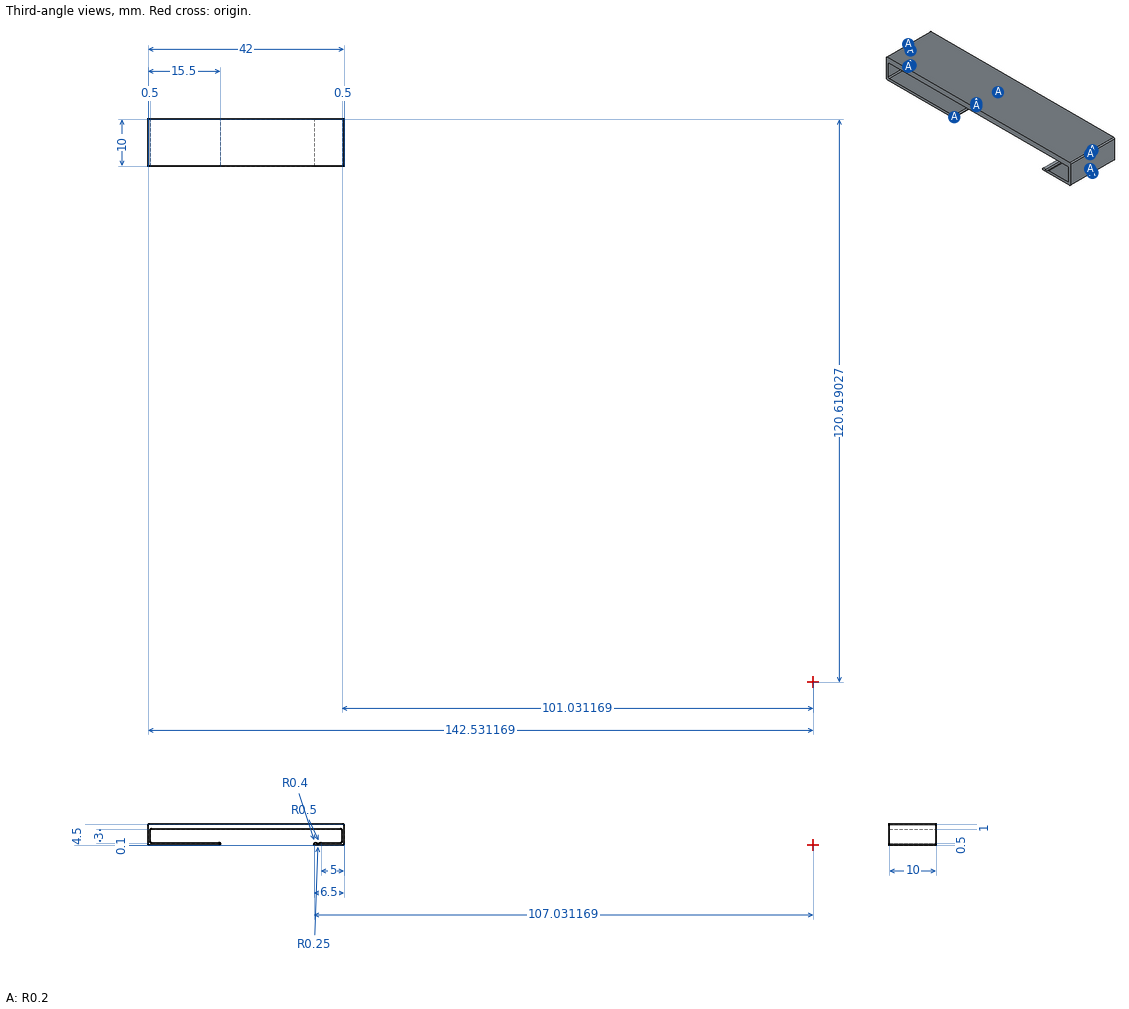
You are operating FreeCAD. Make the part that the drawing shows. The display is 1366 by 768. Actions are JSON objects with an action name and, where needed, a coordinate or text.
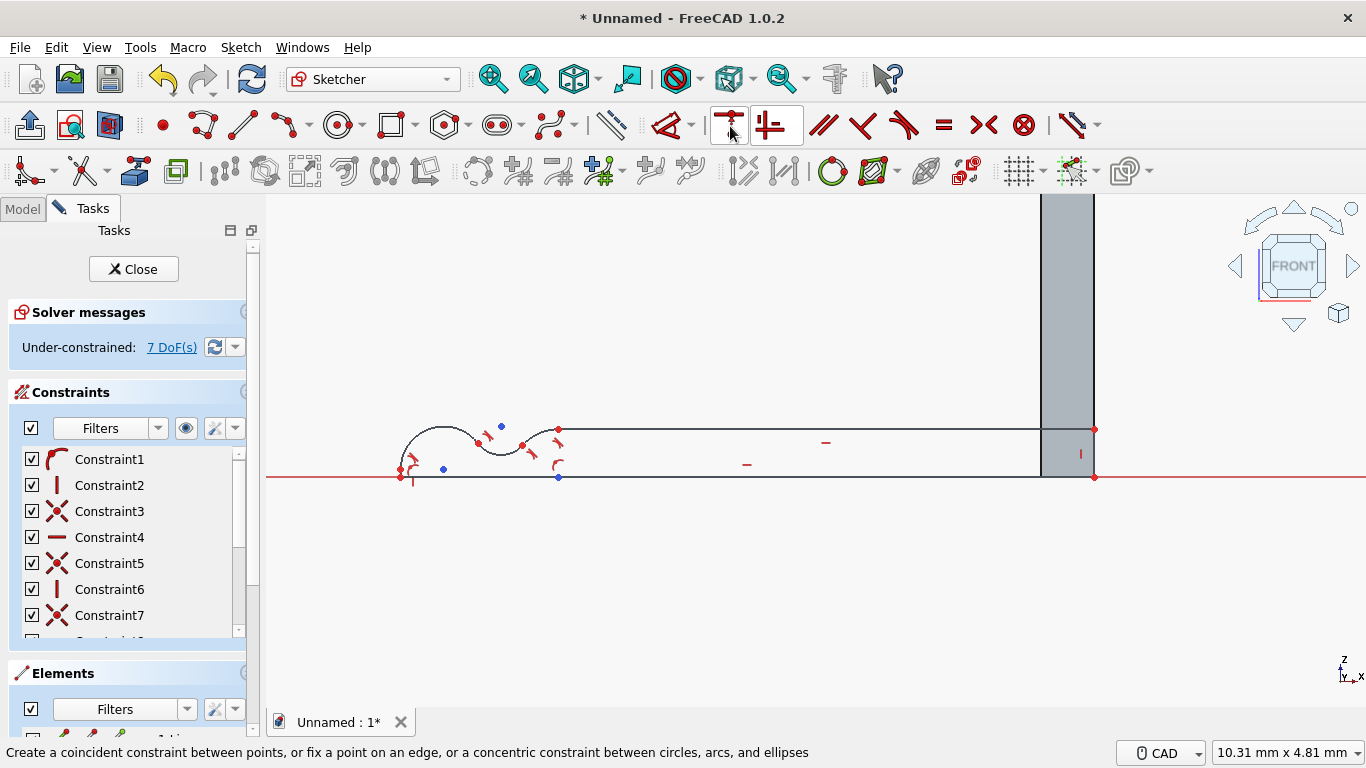
{"action": "left_click", "coordinate": [666, 126]}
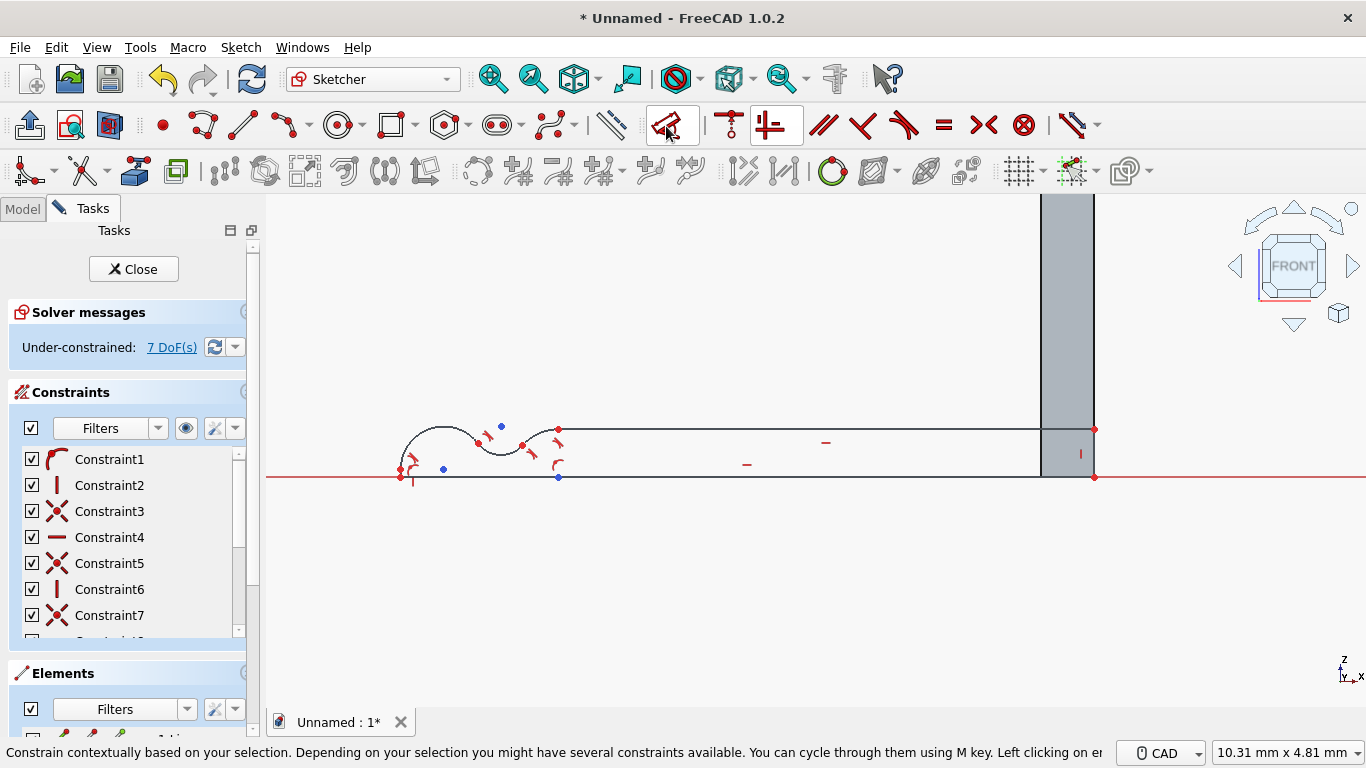
{"action": "left_click", "coordinate": [546, 431]}
{"action": "left_click", "coordinate": [538, 400]}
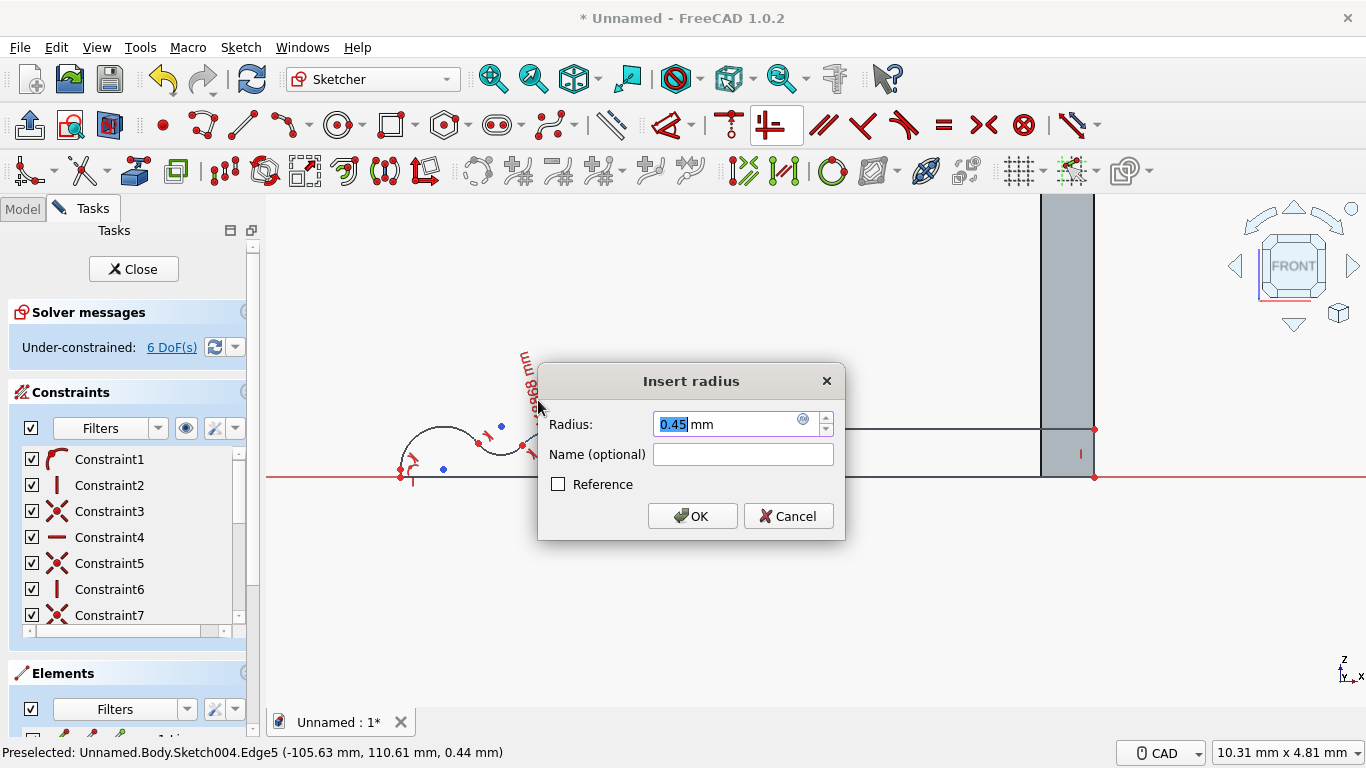
{"action": "type", "text": "0.5"}
{"action": "key", "text": "Return"}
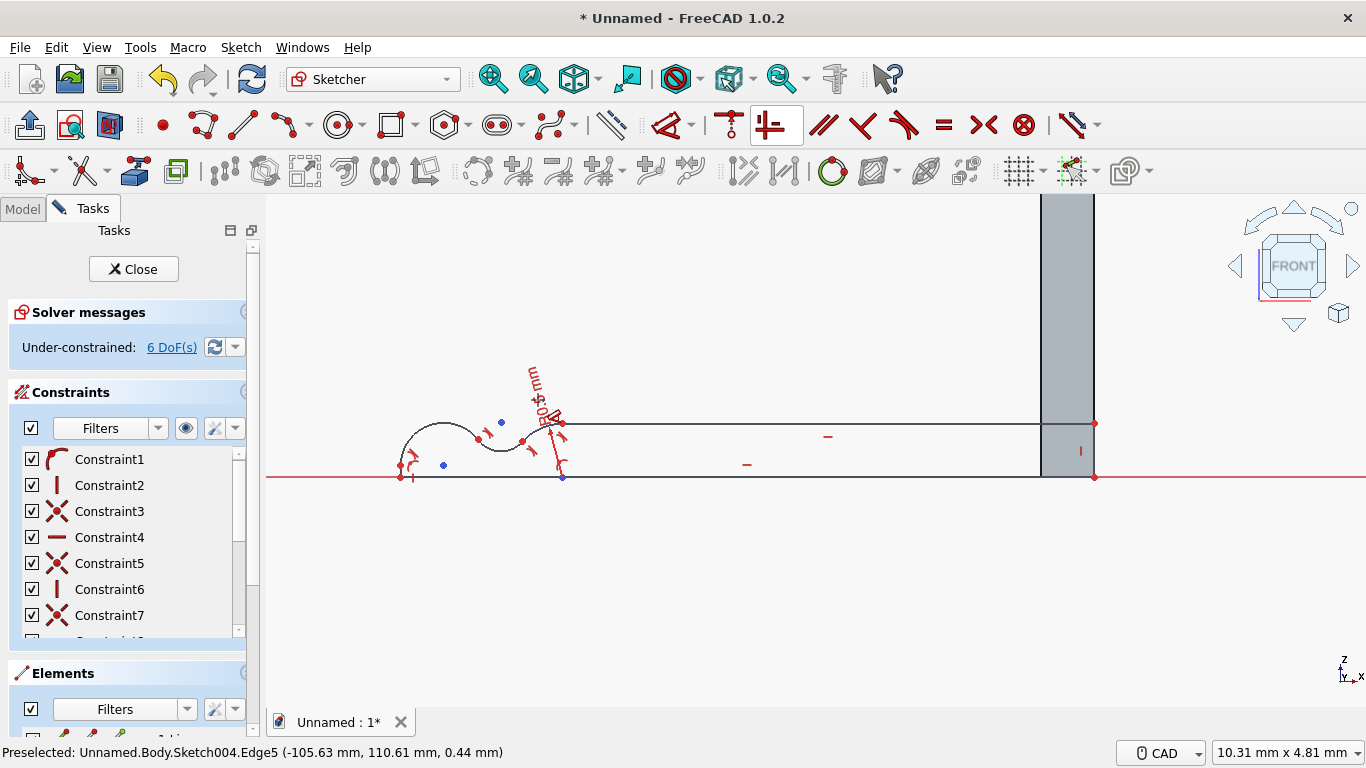
{"action": "scroll", "coordinate": [490, 449], "scroll_direction": "up", "scroll_amount": 2}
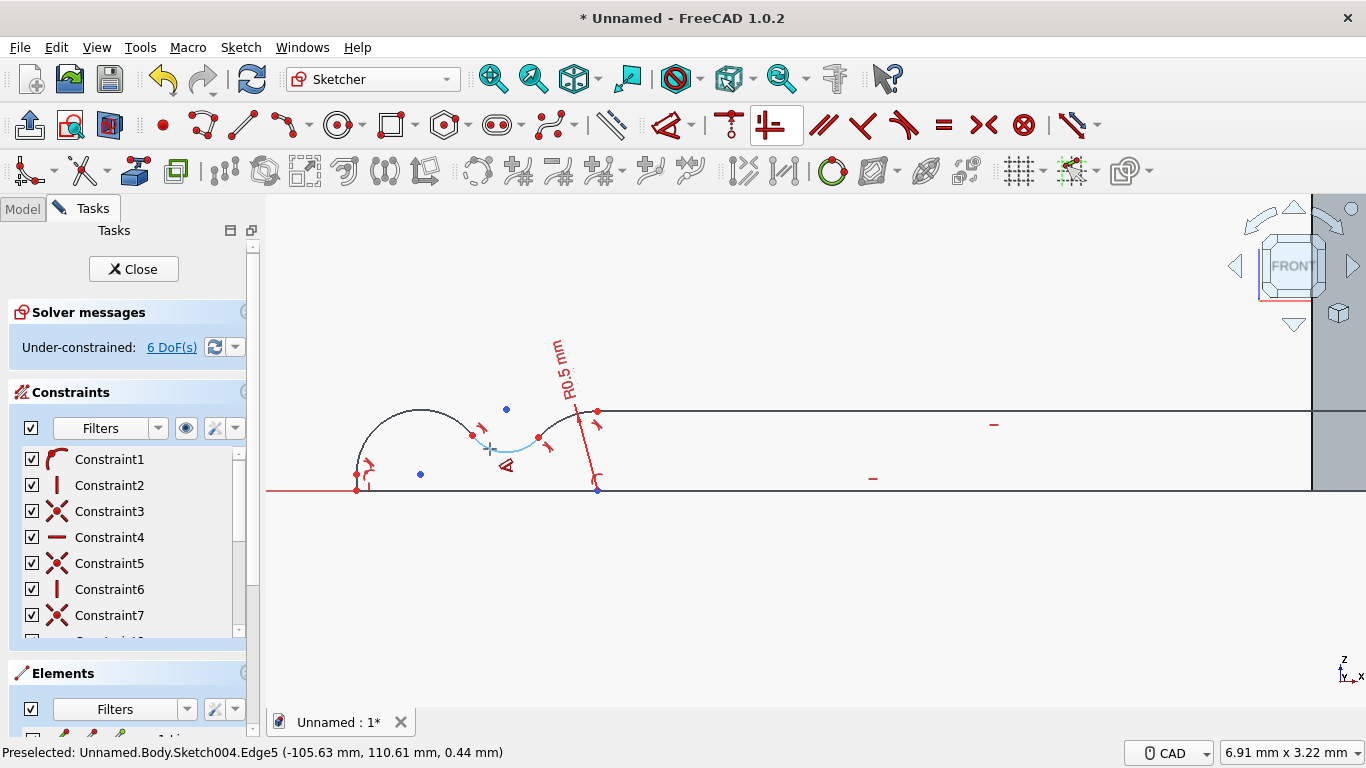
{"action": "left_click", "coordinate": [490, 449]}
{"action": "left_click", "coordinate": [448, 456]}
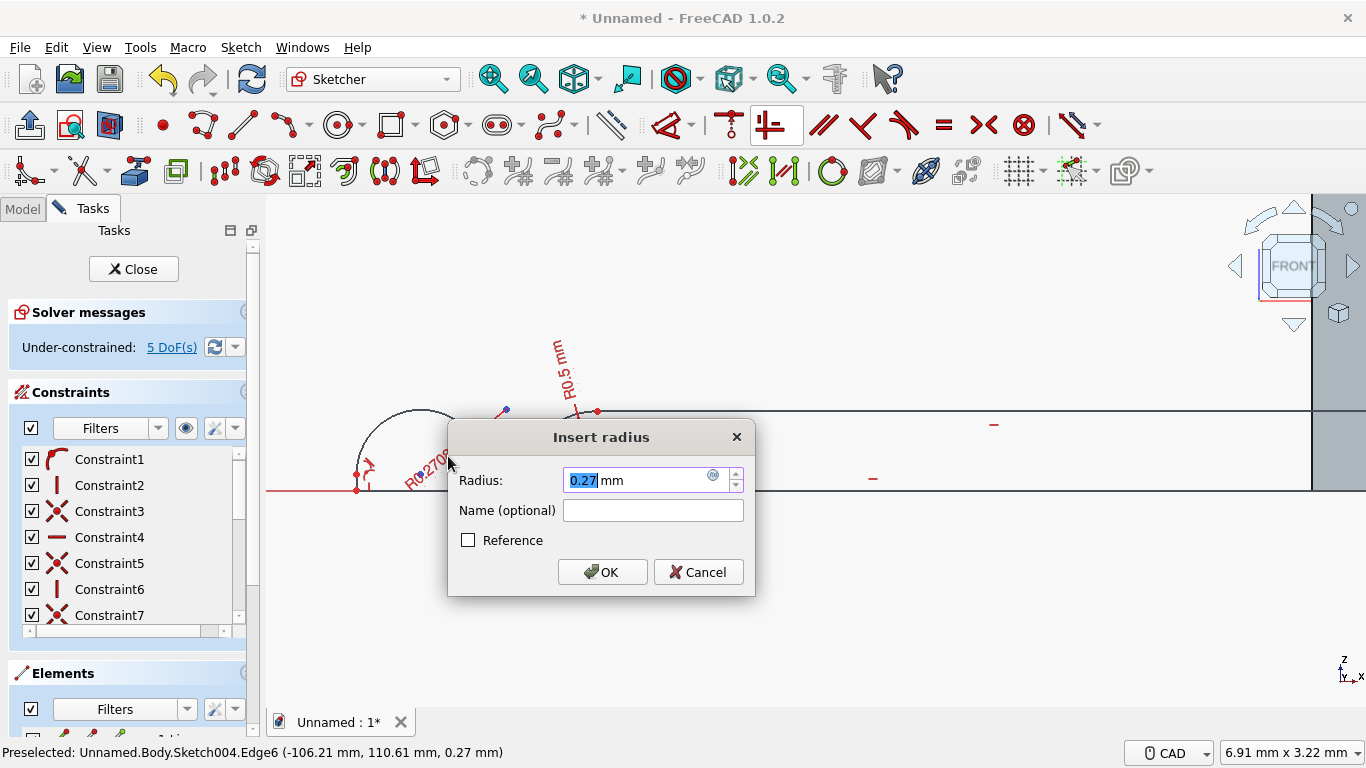
{"action": "type", "text": "0.25"}
{"action": "key", "text": "Return"}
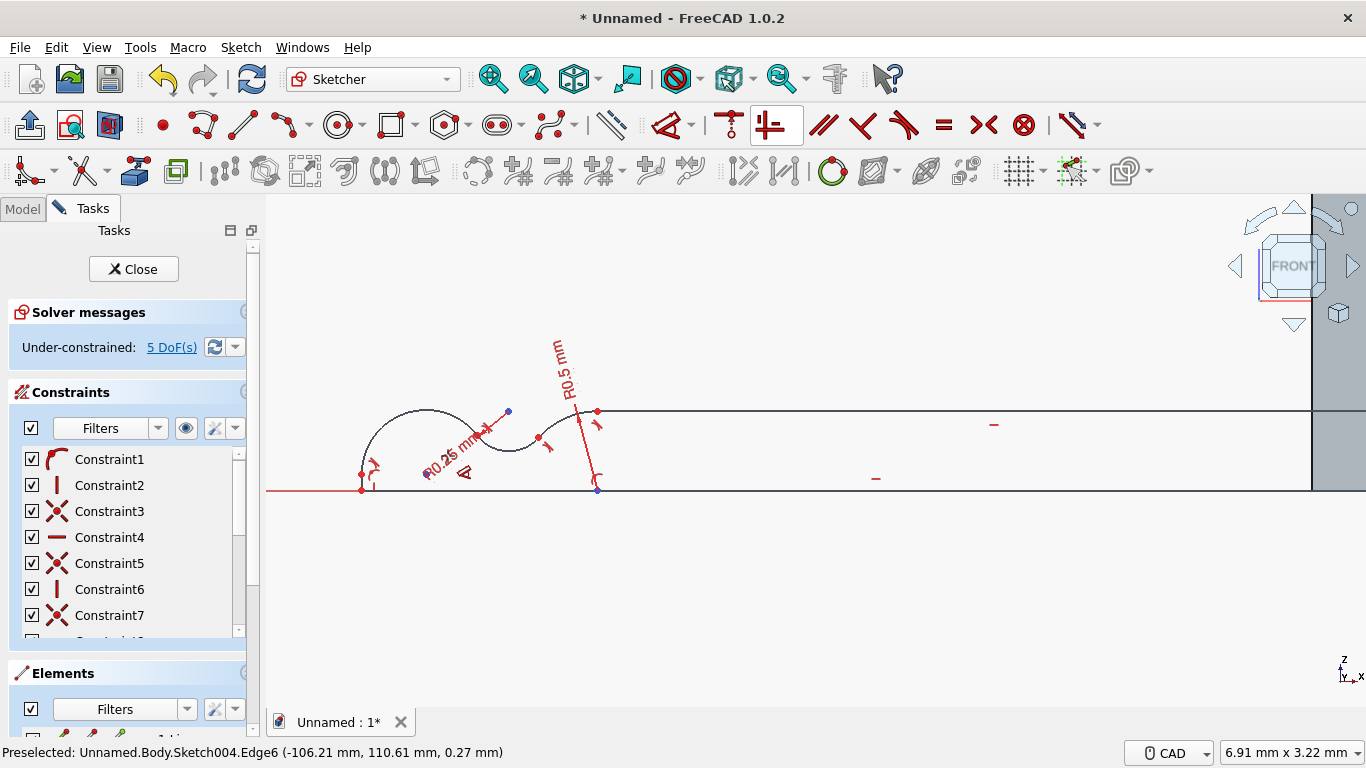
{"action": "left_click", "coordinate": [437, 411]}
{"action": "left_click", "coordinate": [442, 379]}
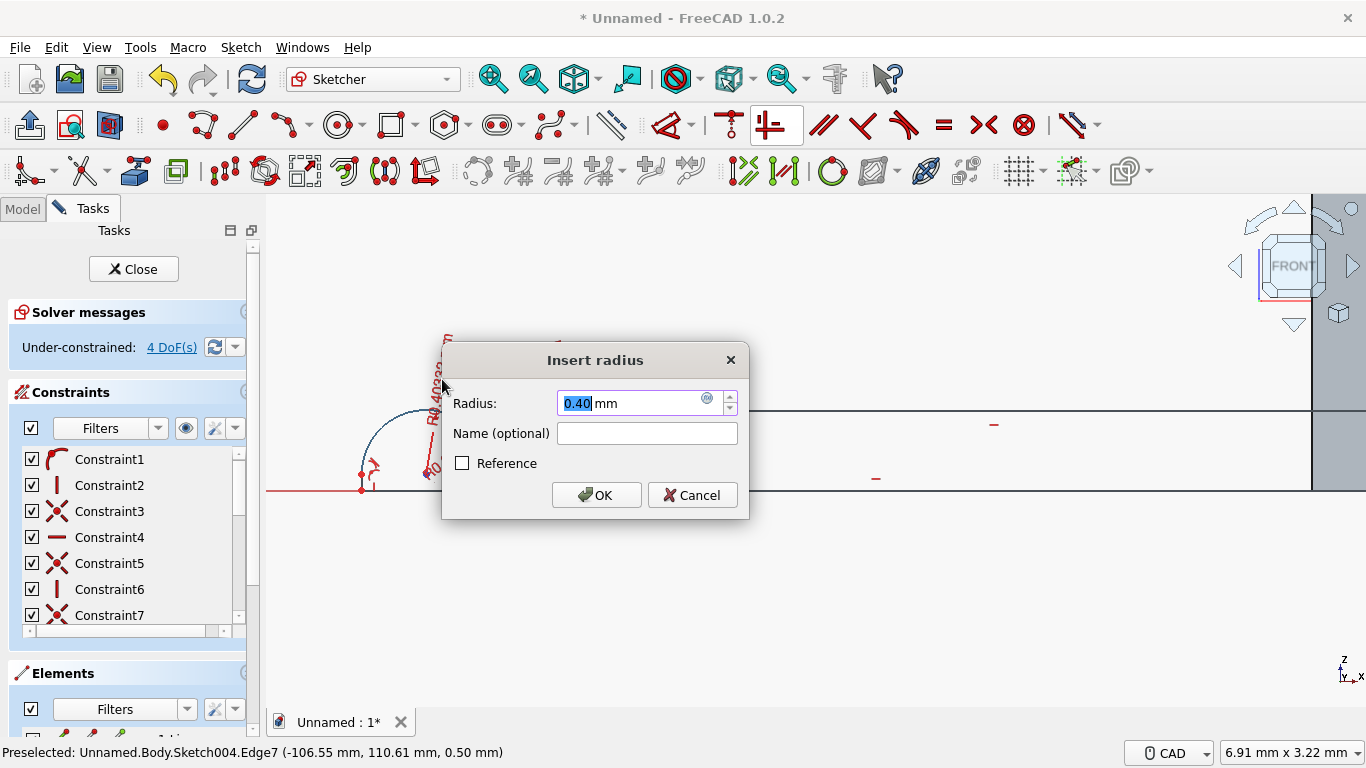
{"action": "type", "text": "0.4"}
{"action": "key", "text": "Return"}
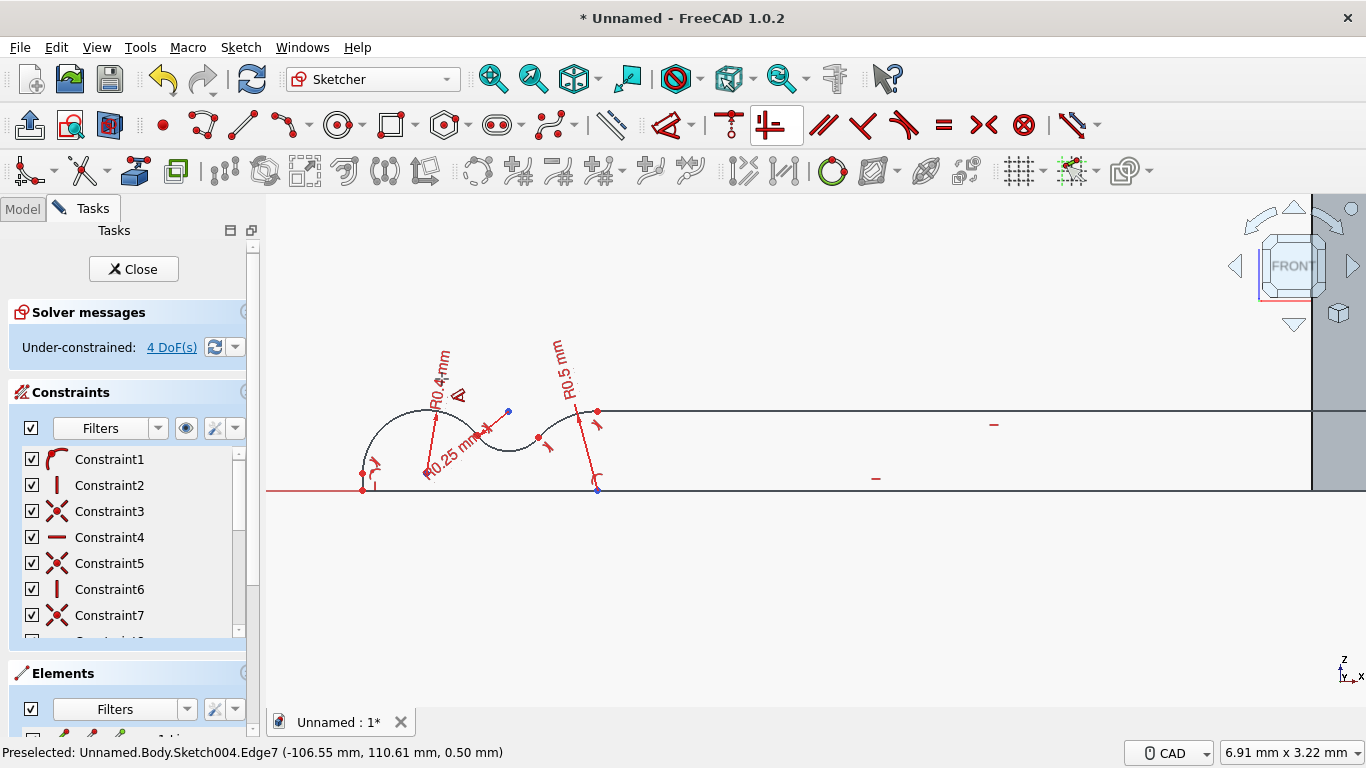
{"action": "left_click", "coordinate": [1153, 411]}
{"action": "left_click", "coordinate": [899, 377]}